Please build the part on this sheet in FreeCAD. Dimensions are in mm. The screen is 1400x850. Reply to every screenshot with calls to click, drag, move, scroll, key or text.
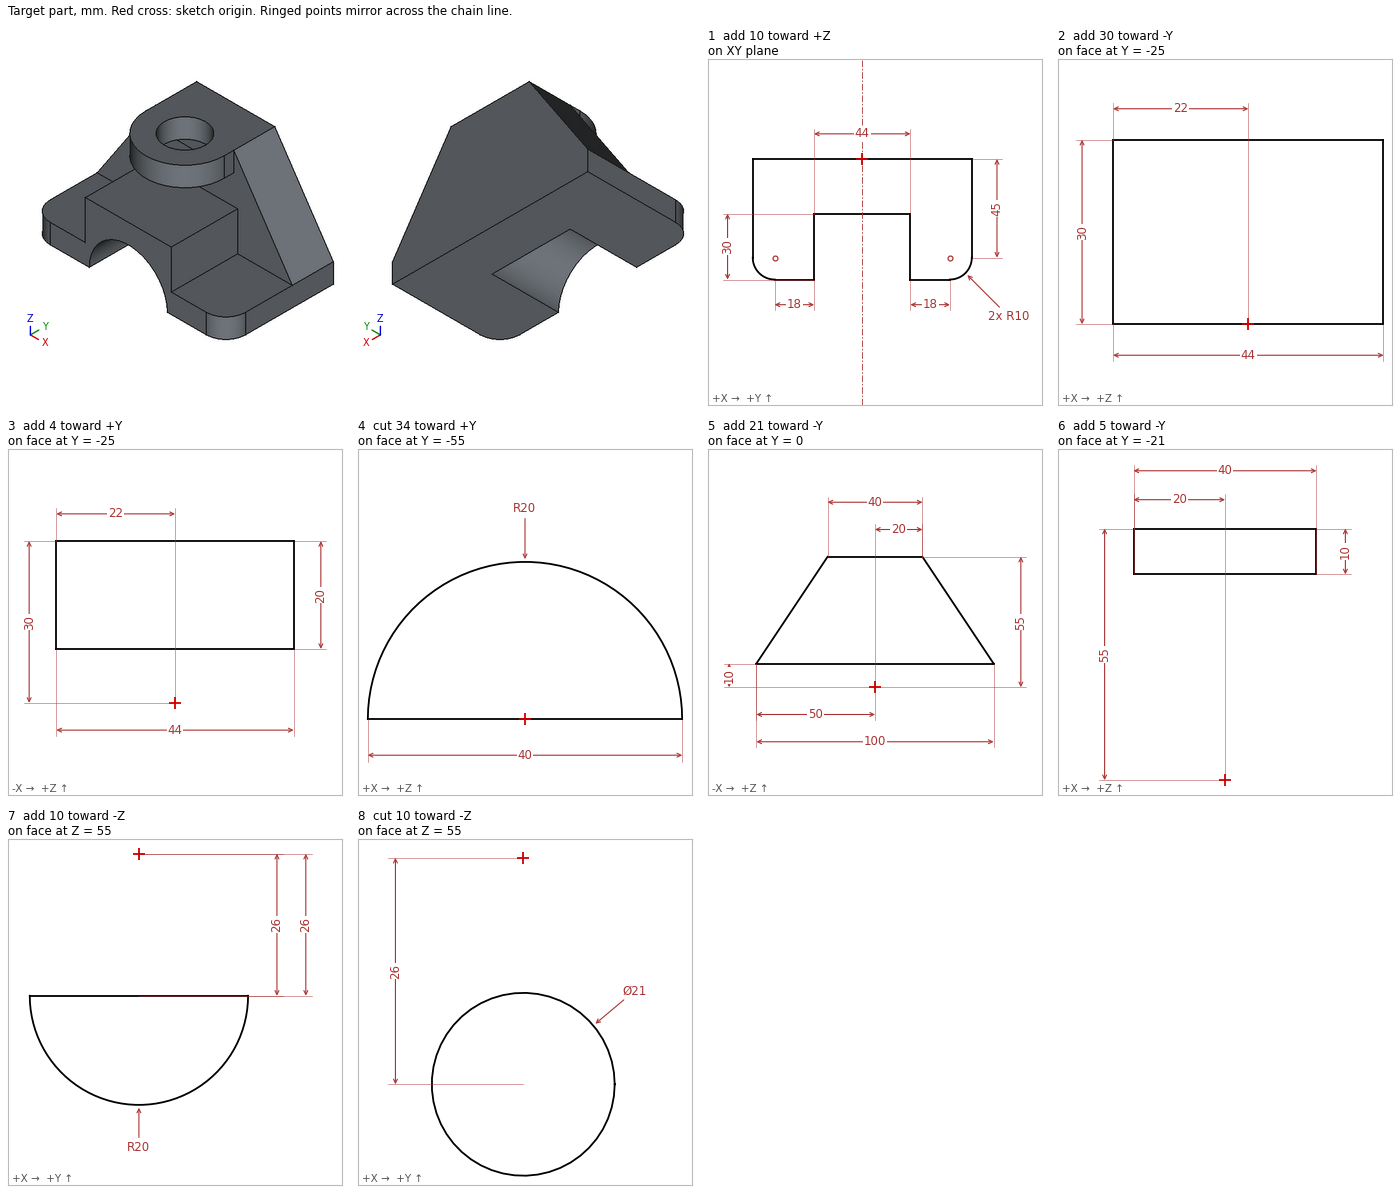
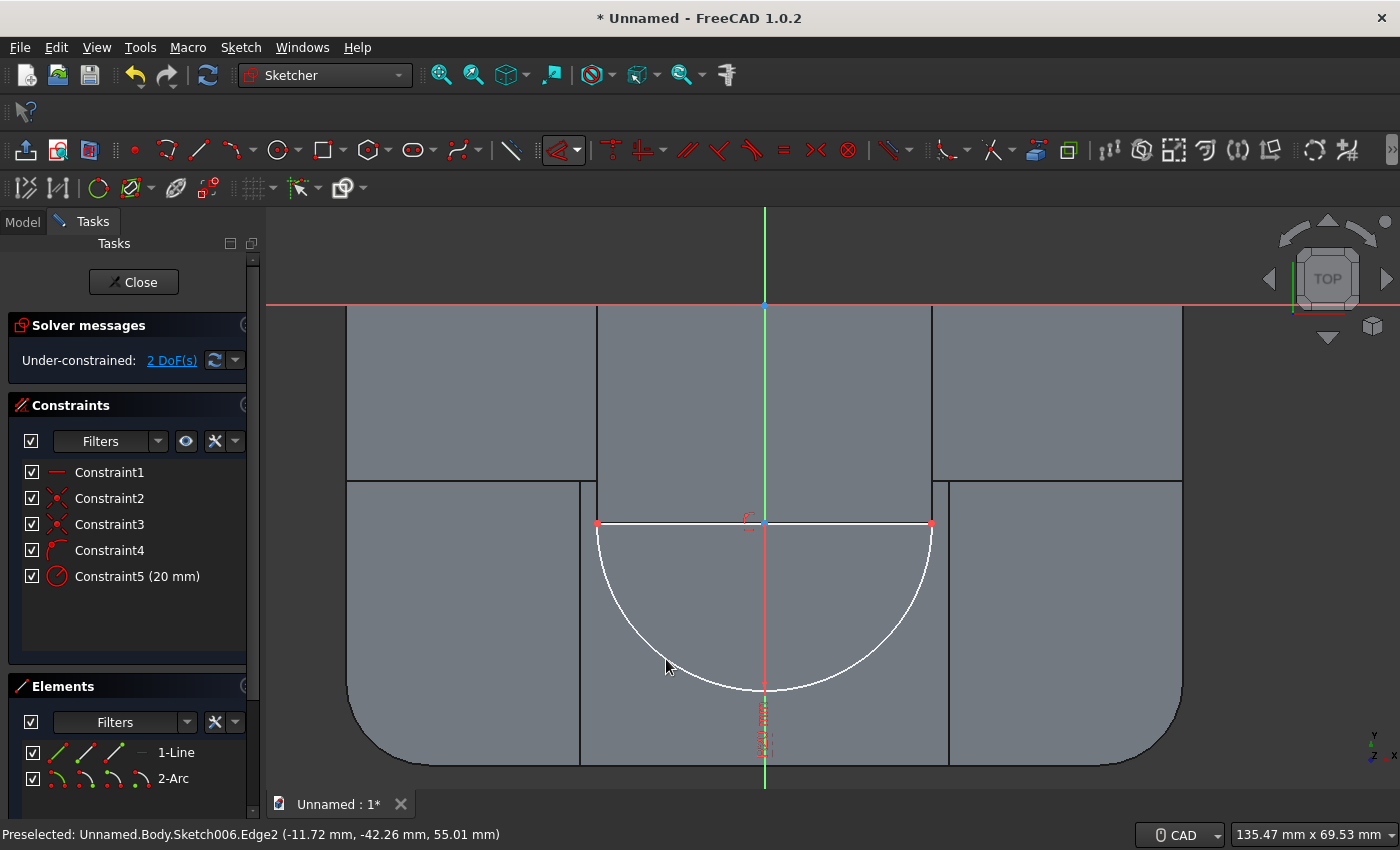
click(932, 524)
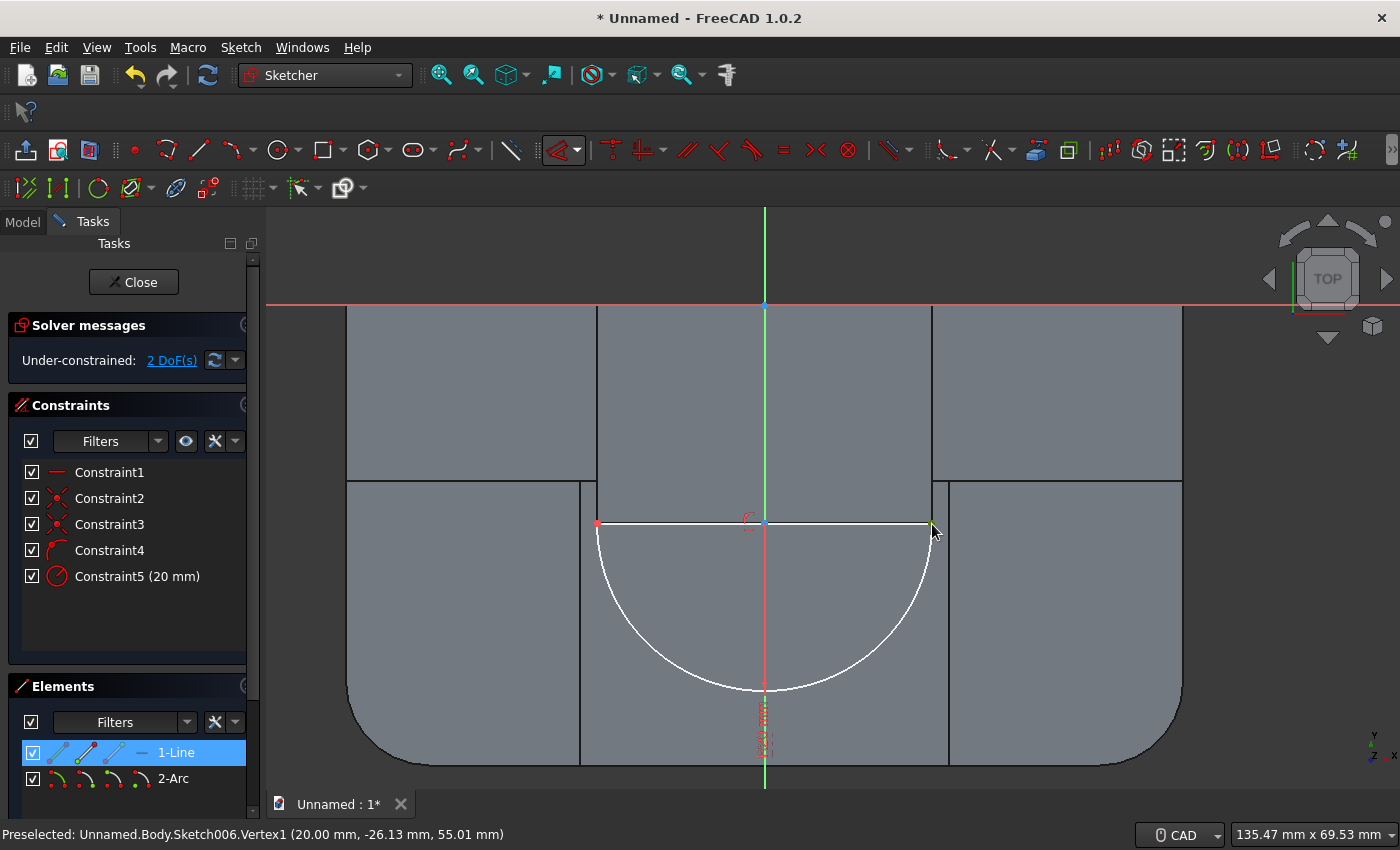
key(i)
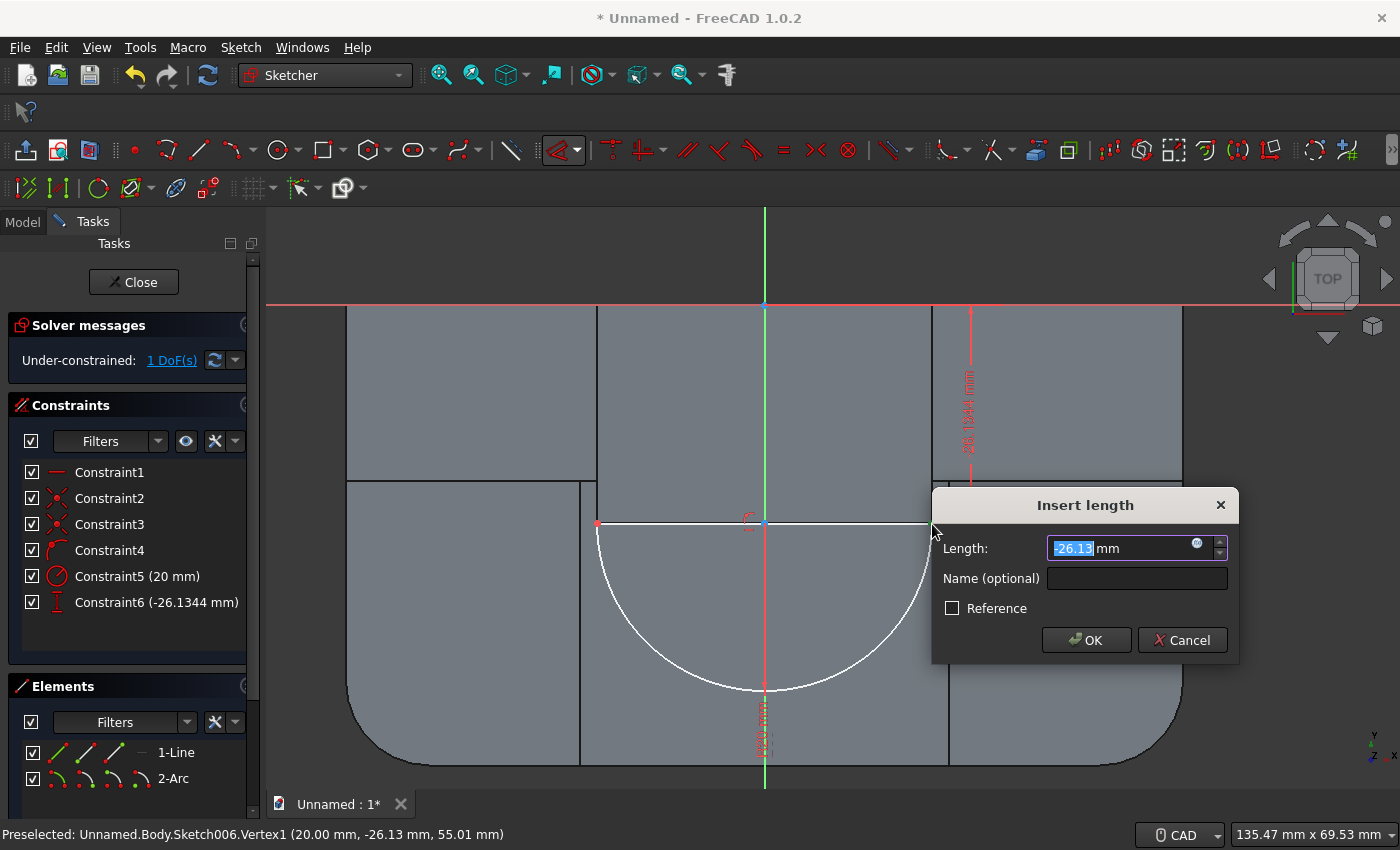
text(-26)
key(Return)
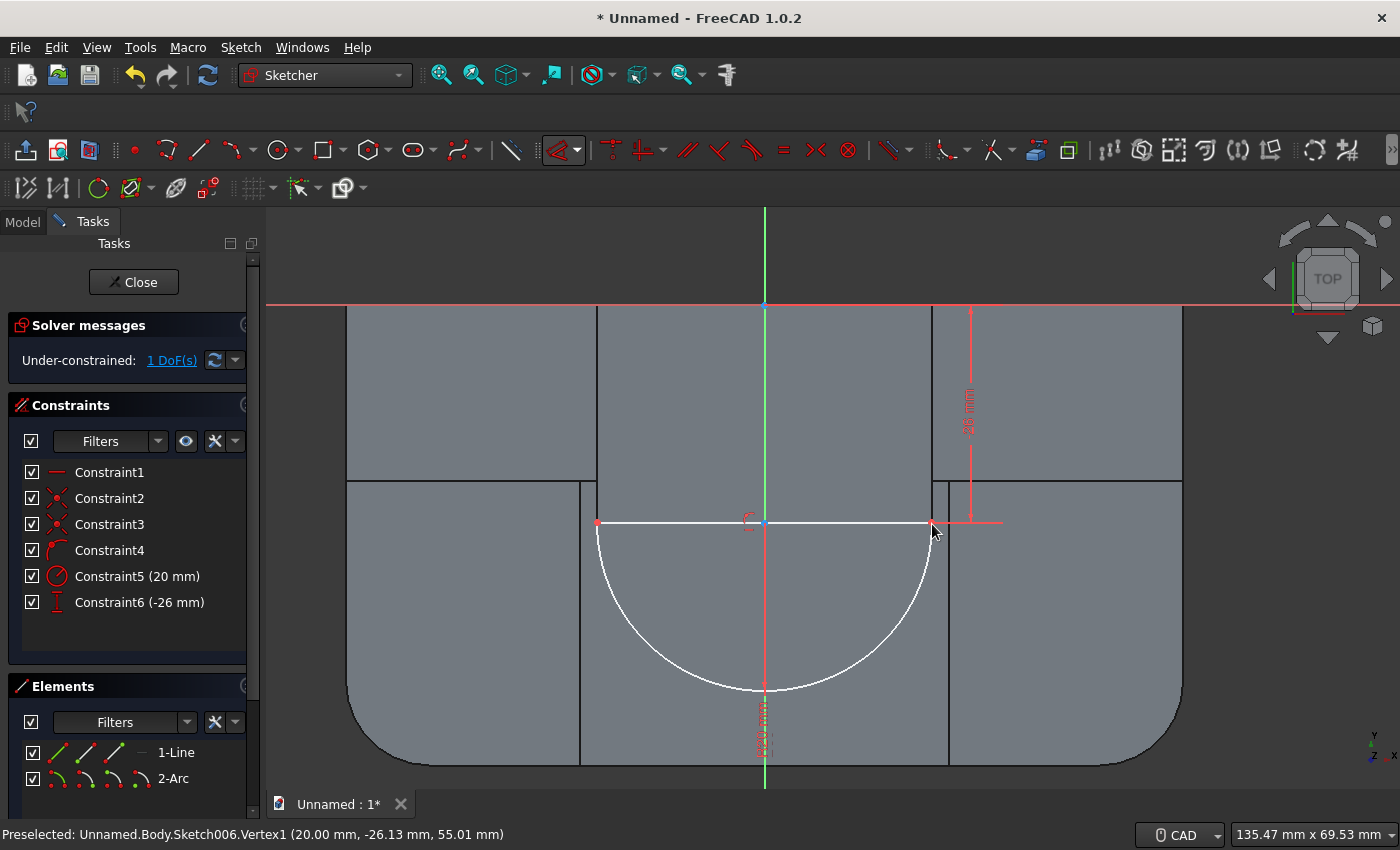
click(765, 524)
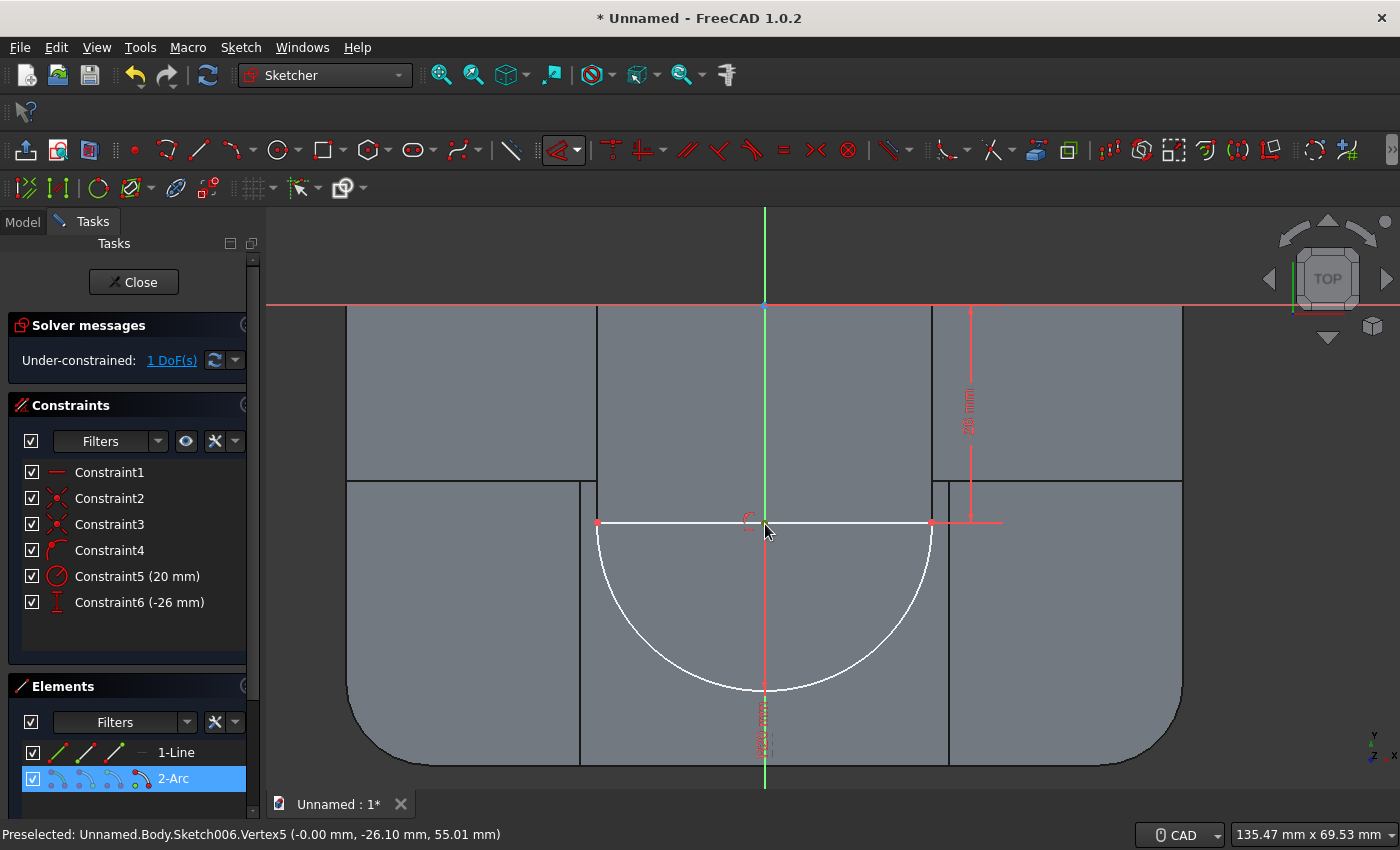
key(i)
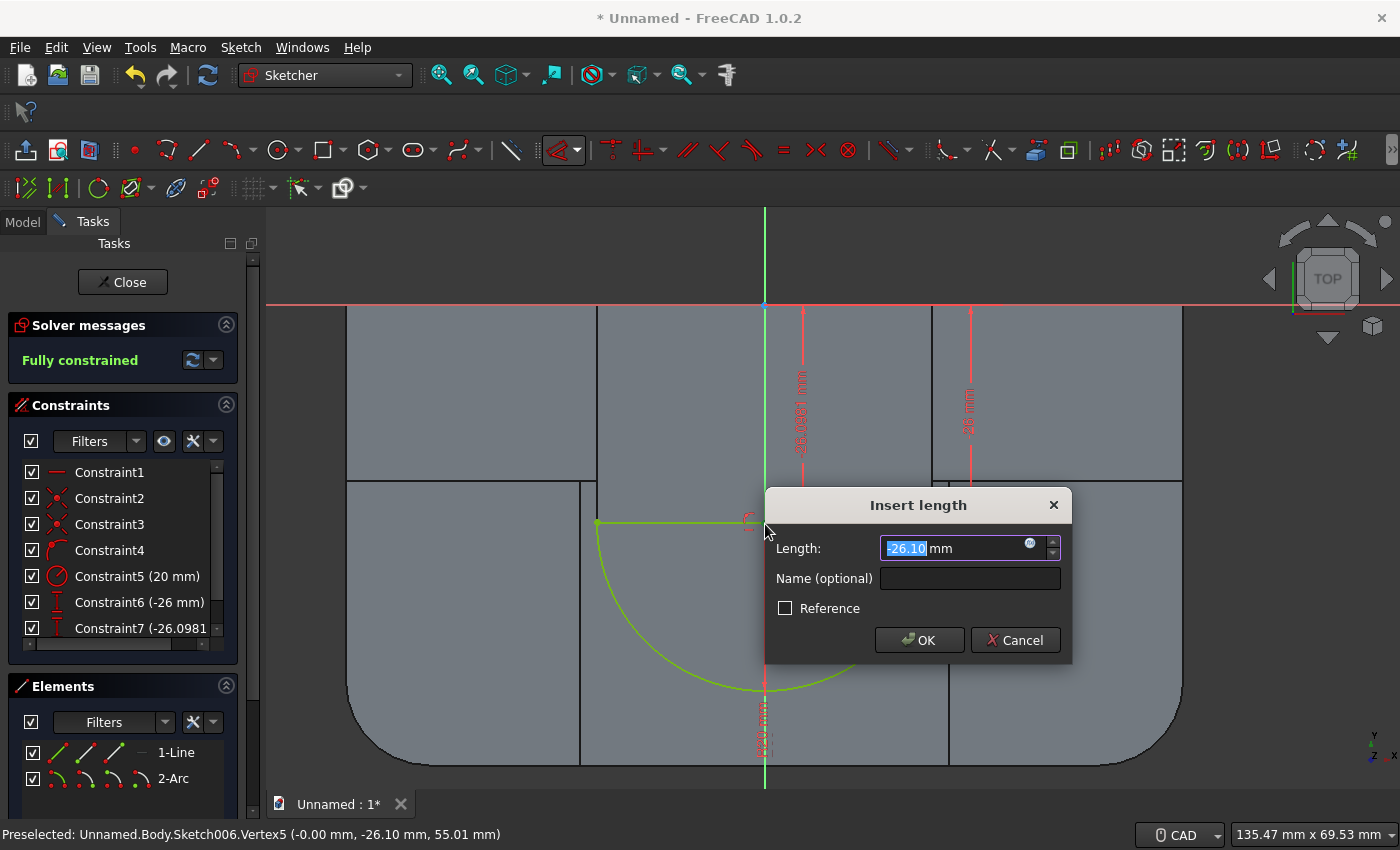
text(-26)
key(Return)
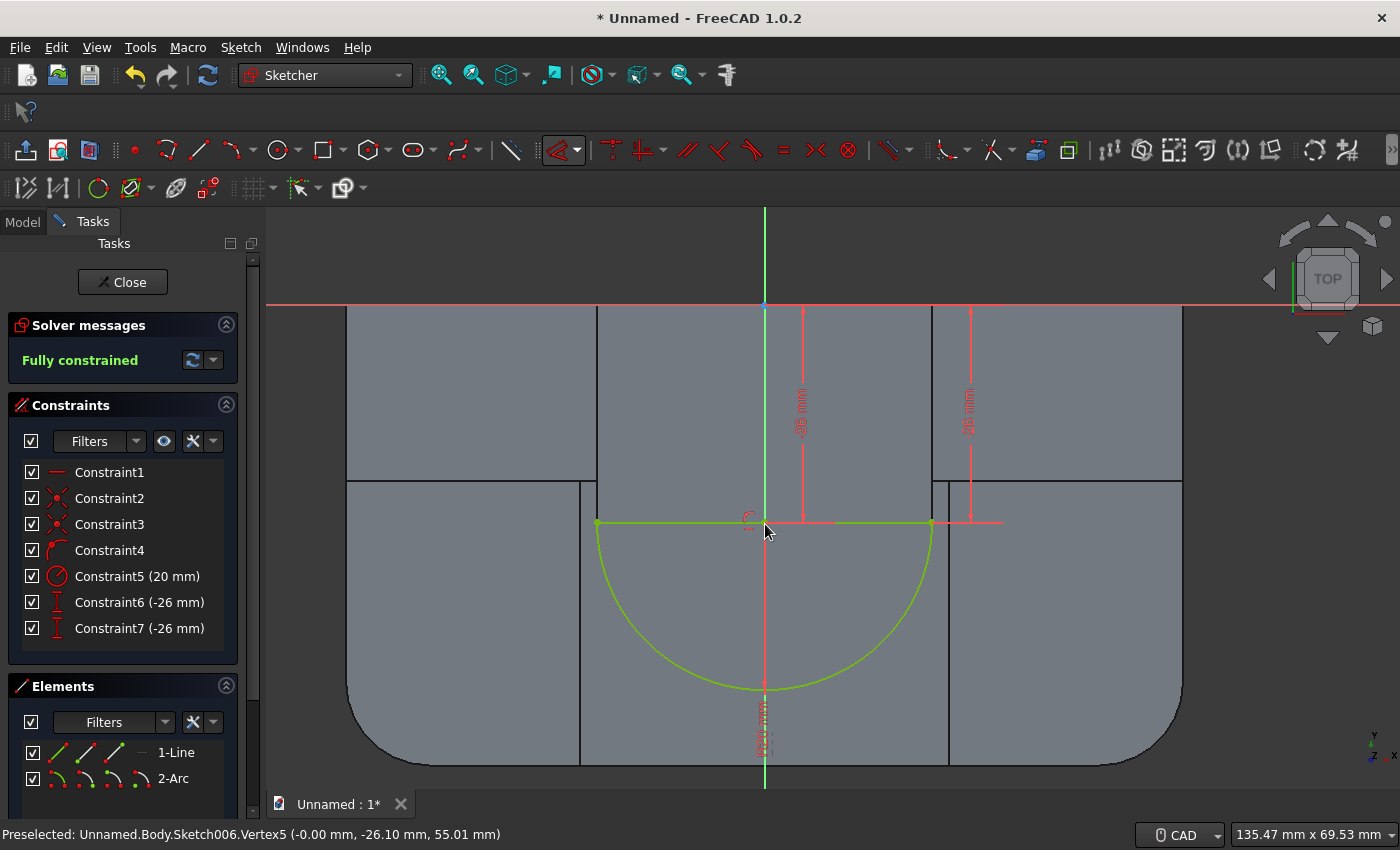
click(123, 282)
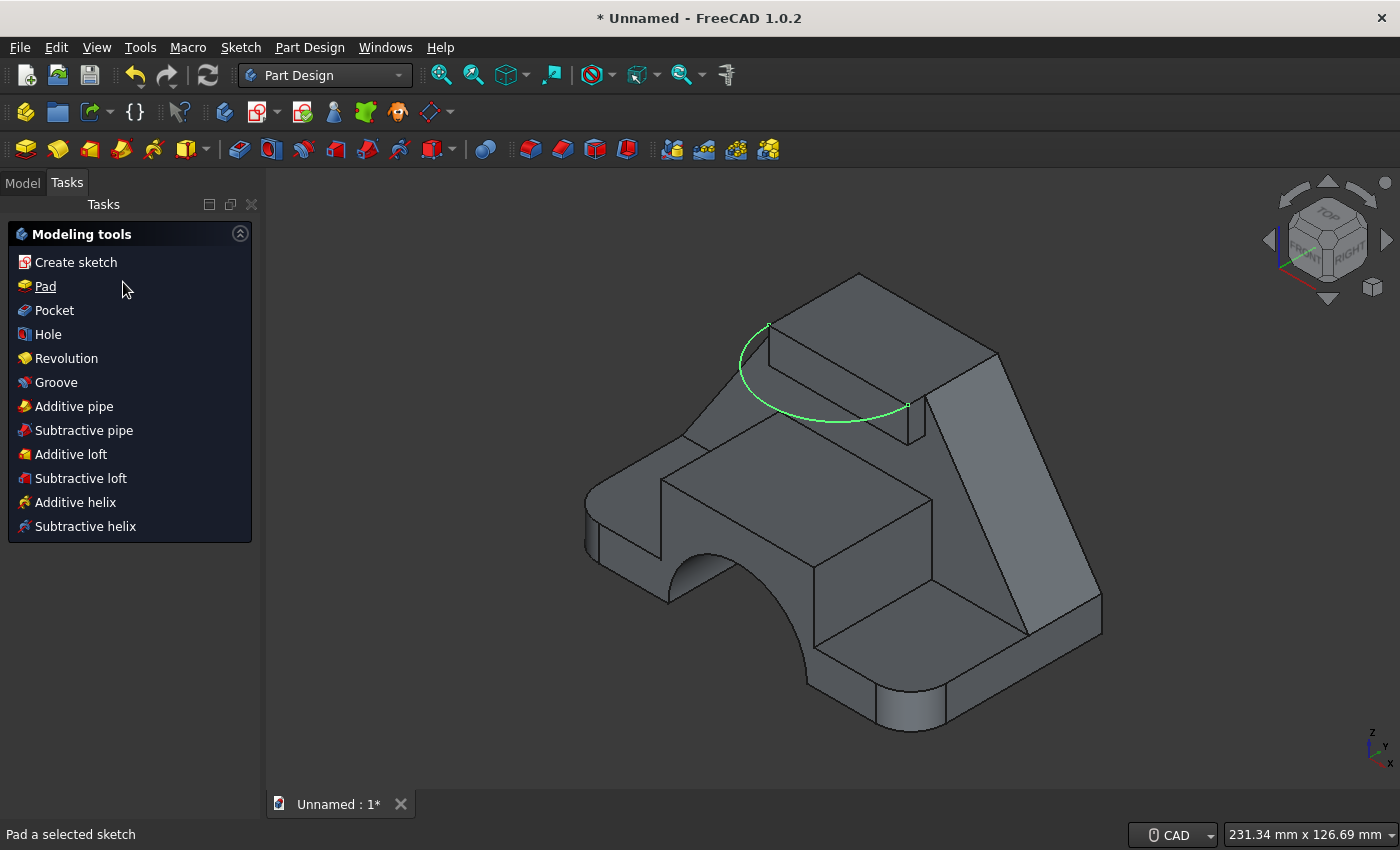
click(26, 150)